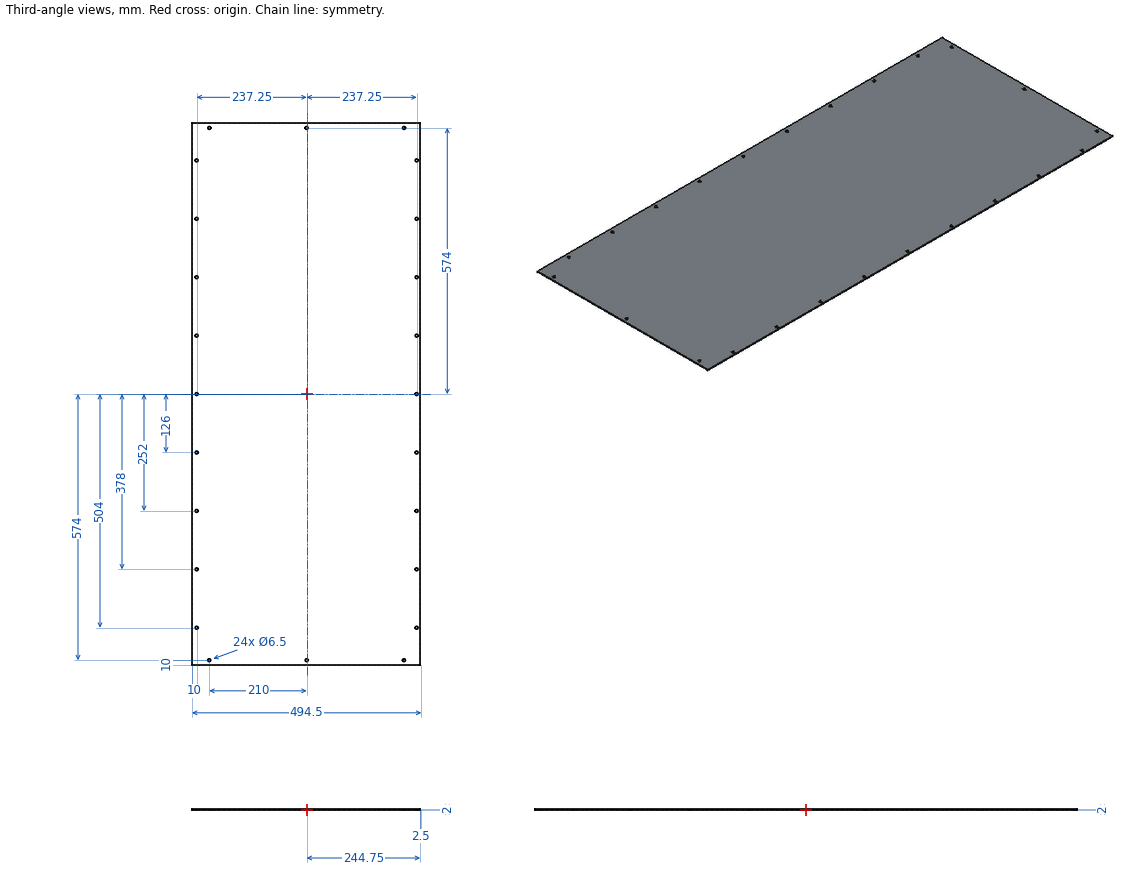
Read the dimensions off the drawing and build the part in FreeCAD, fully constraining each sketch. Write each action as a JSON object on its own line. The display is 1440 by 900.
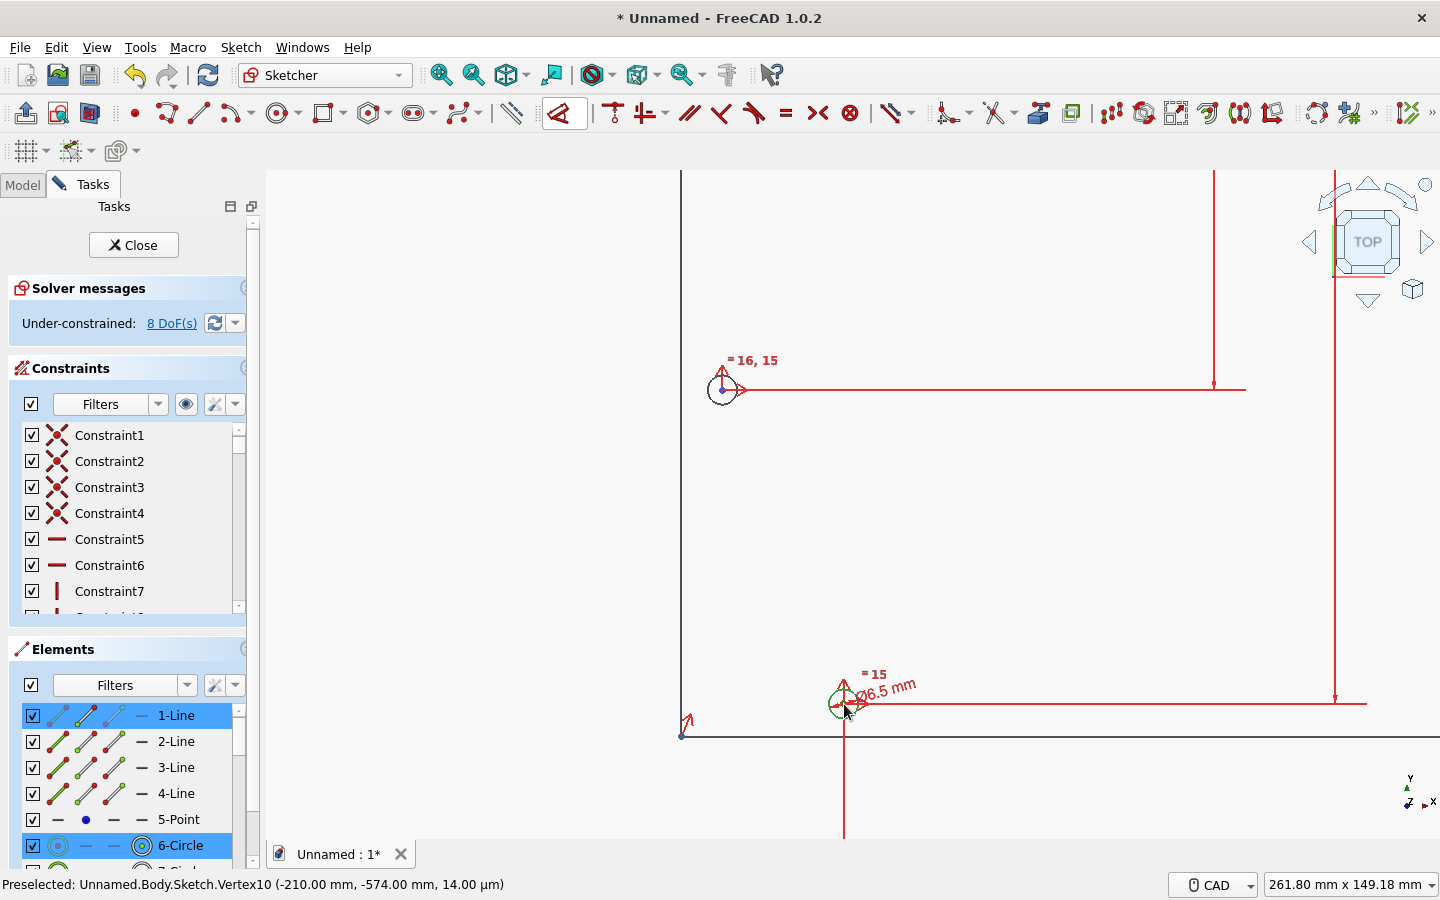
{"action": "left_click", "coordinate": [582, 114]}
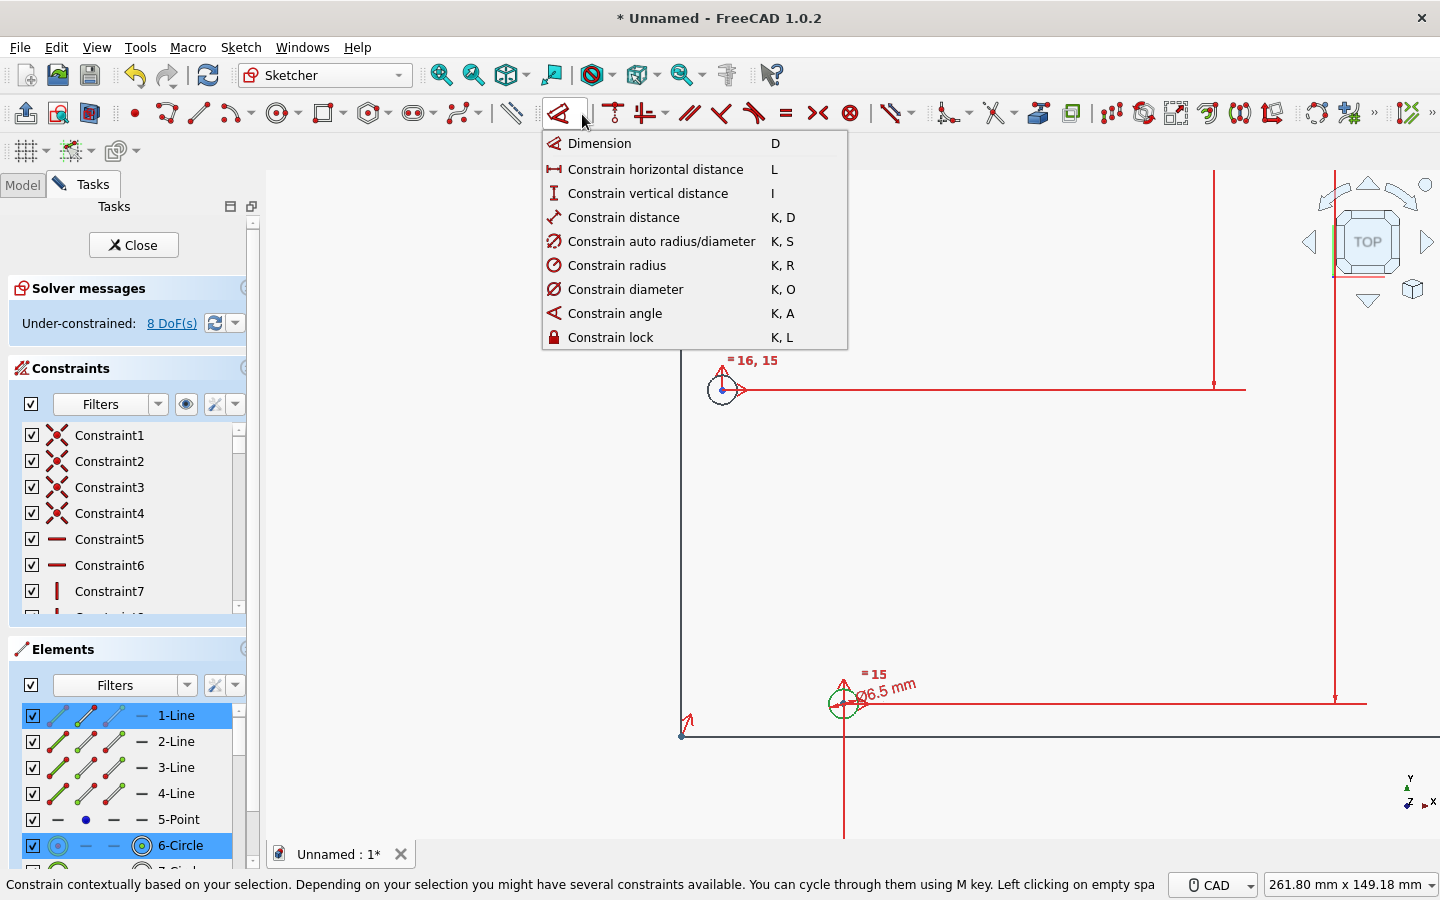
{"action": "left_click", "coordinate": [695, 193]}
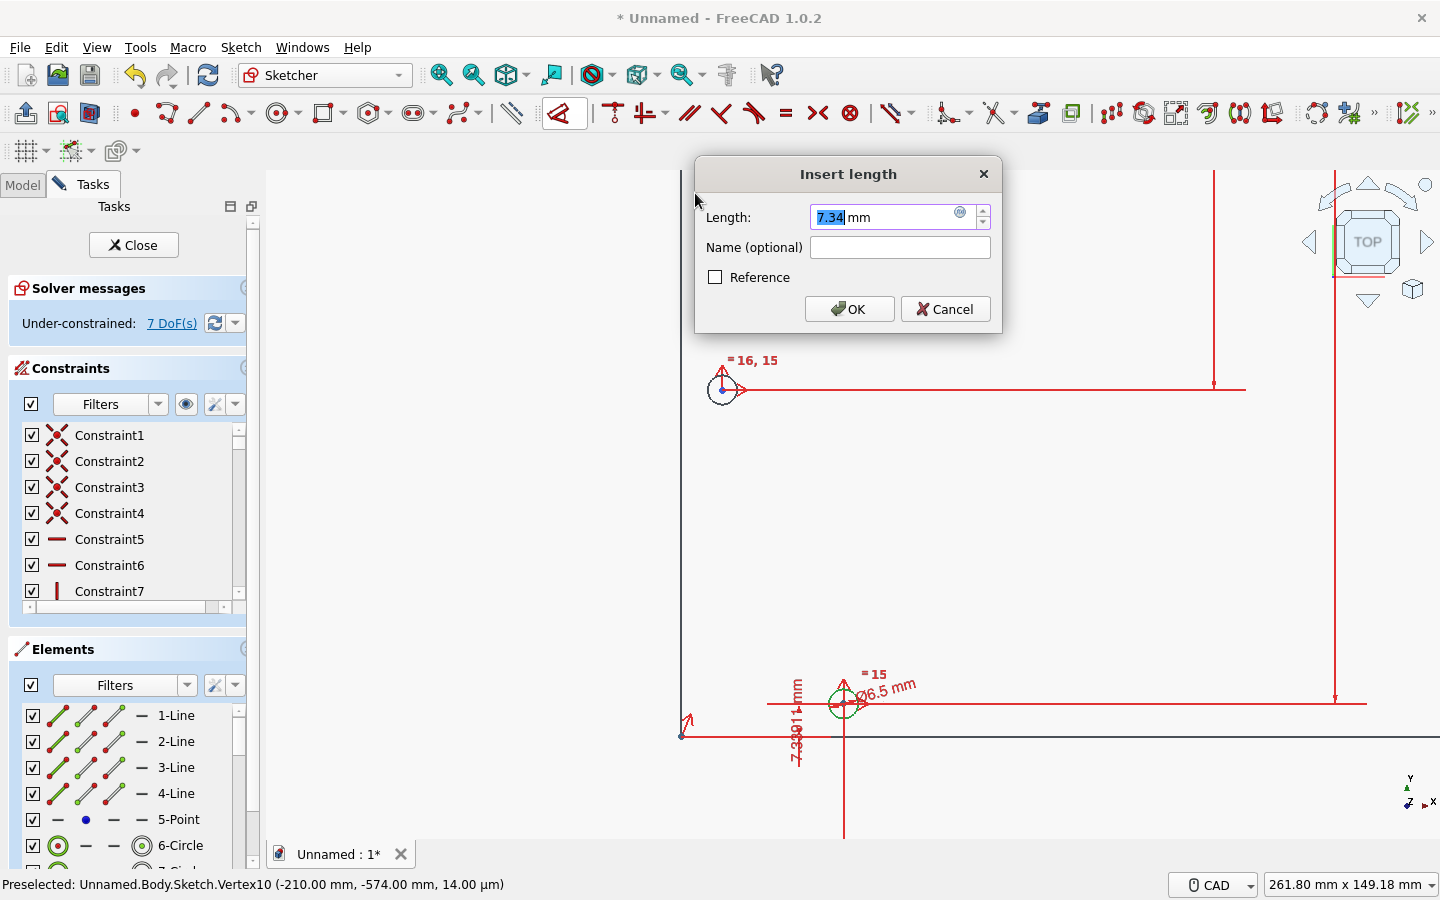
{"action": "type", "text": "10"}
{"action": "key", "text": "Return"}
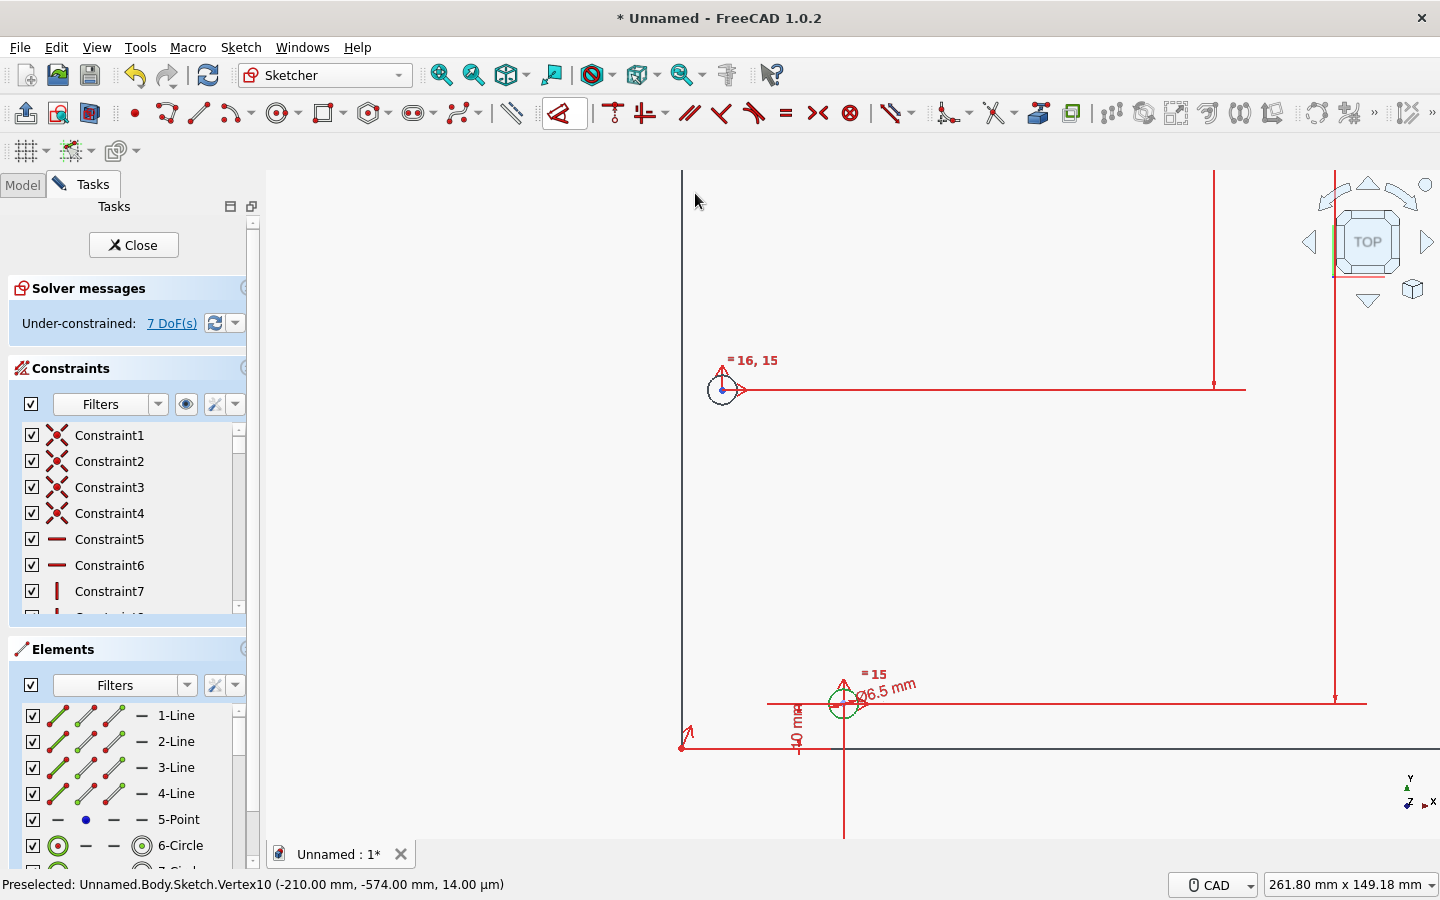
{"action": "left_click", "coordinate": [682, 749]}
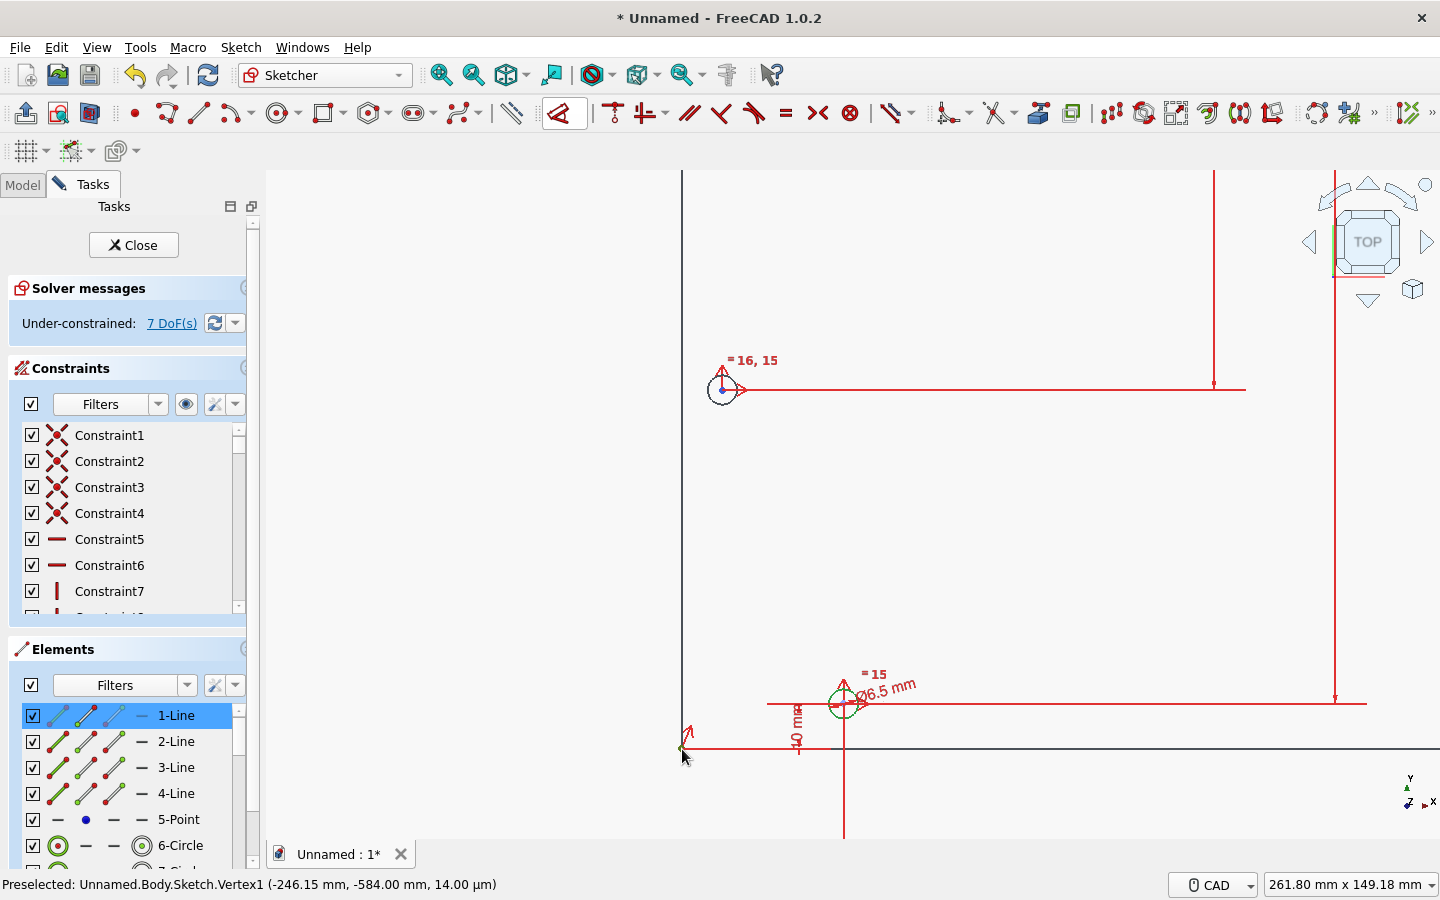
{"action": "left_click", "coordinate": [722, 390]}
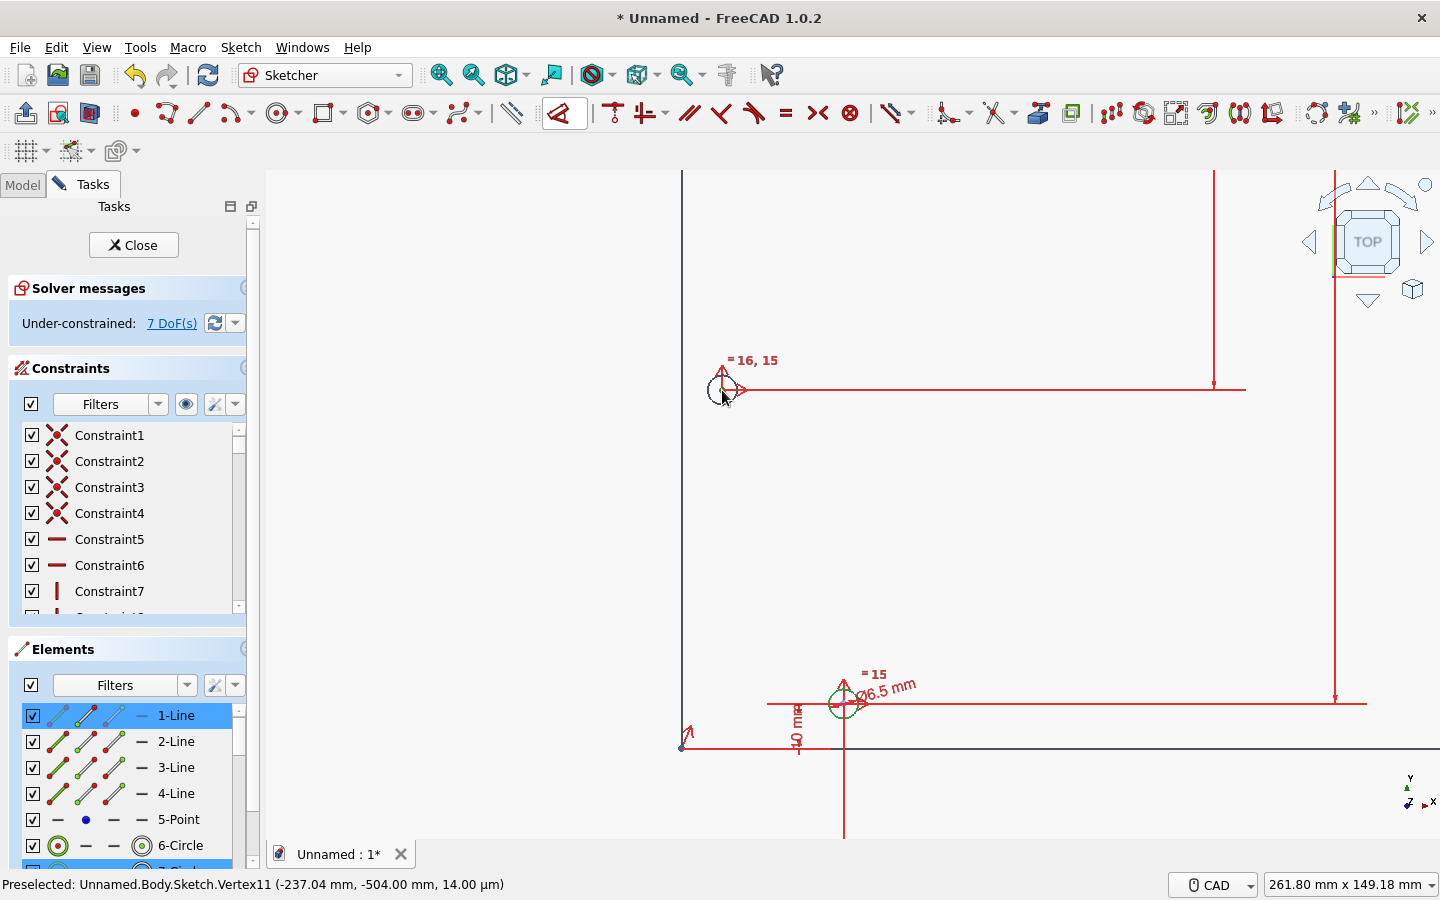
{"action": "left_click", "coordinate": [582, 114]}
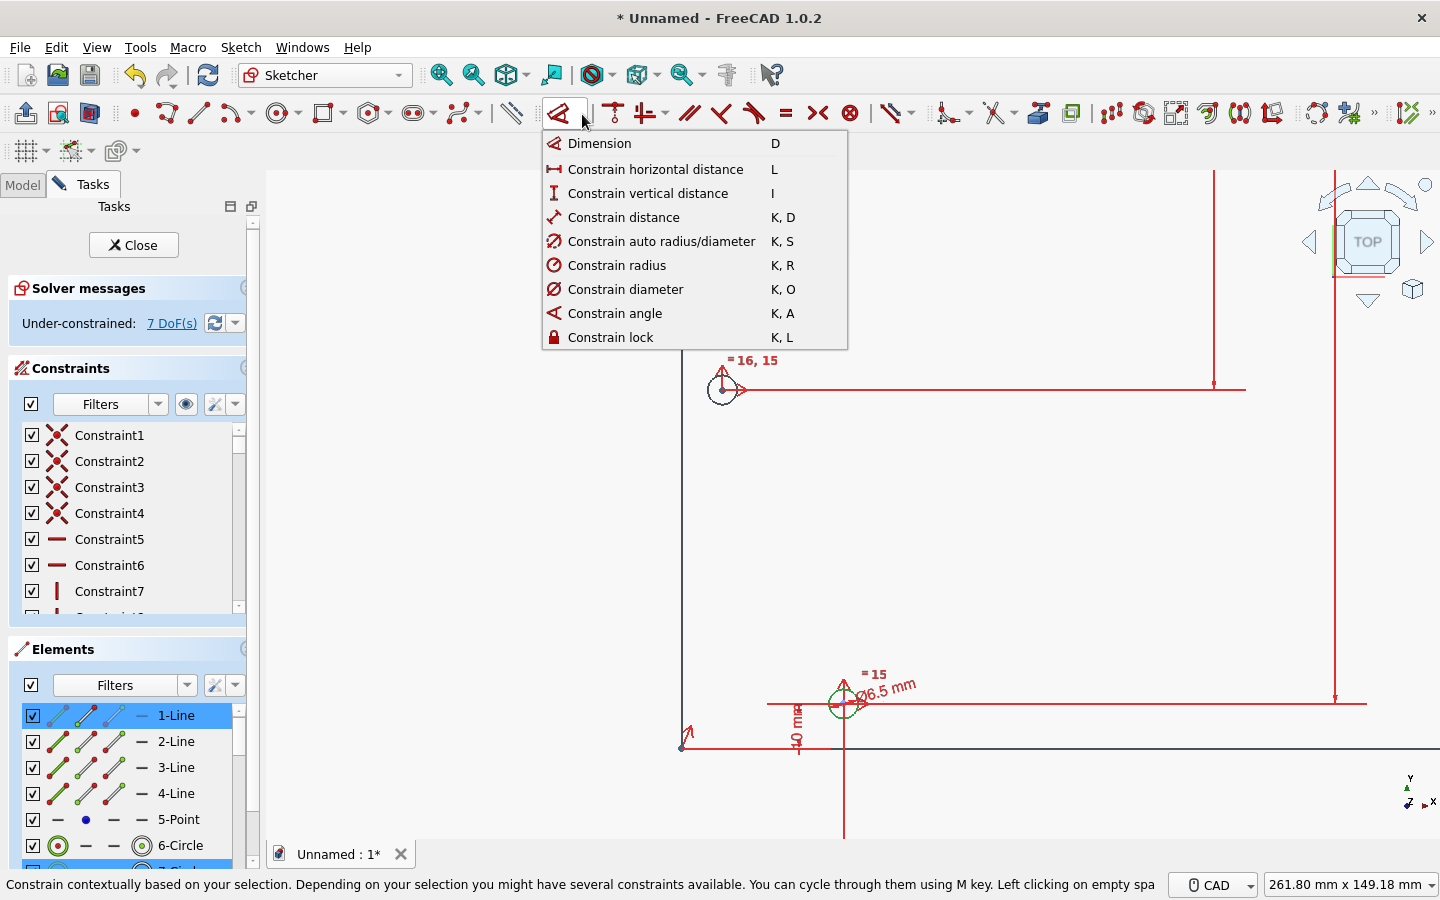
{"action": "left_click", "coordinate": [695, 169]}